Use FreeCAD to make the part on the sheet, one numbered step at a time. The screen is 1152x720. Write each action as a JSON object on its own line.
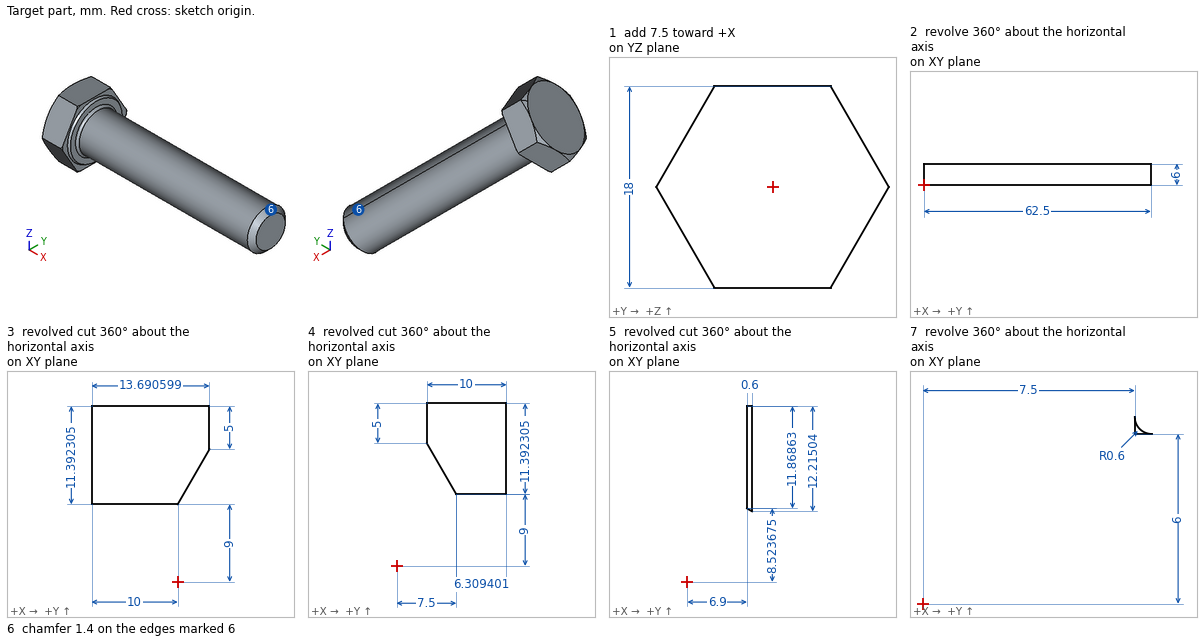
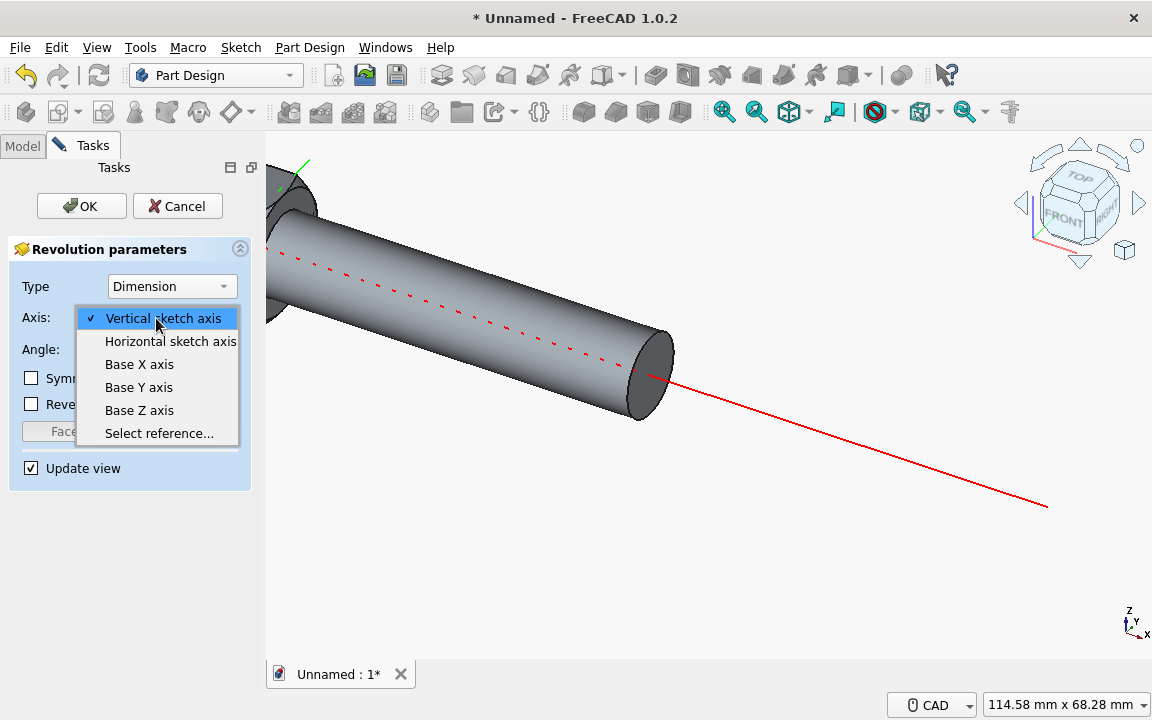
{"action": "left_click", "coordinate": [156, 342]}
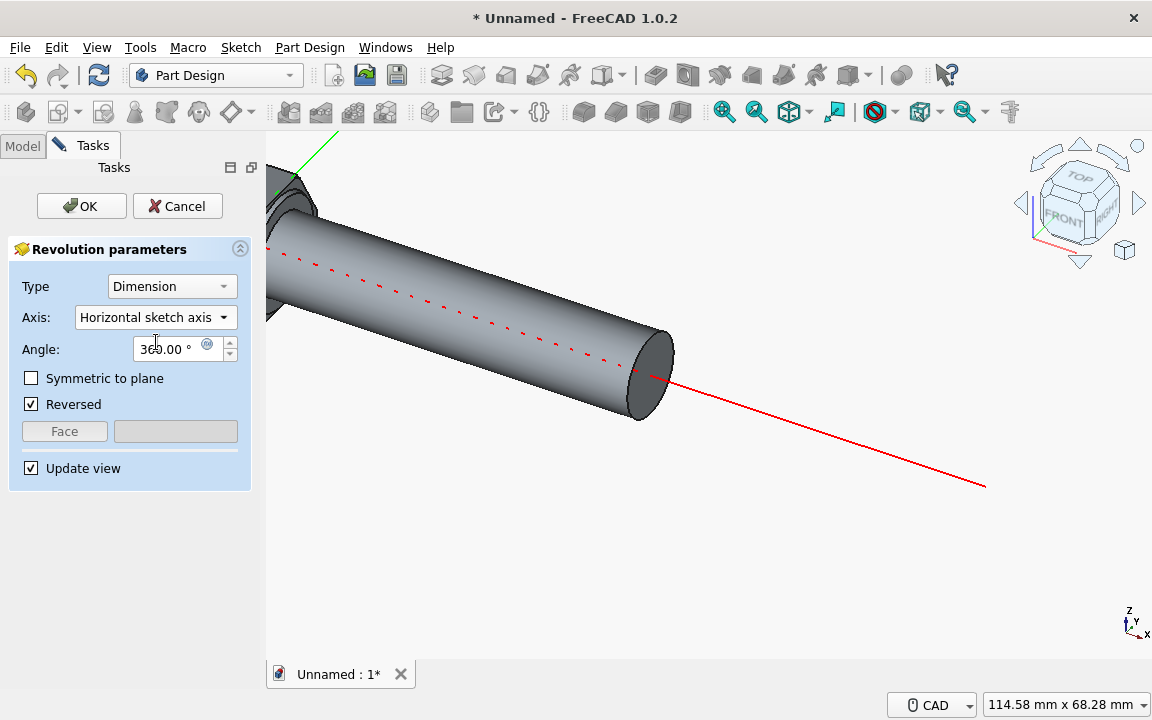
{"action": "left_click", "coordinate": [82, 206]}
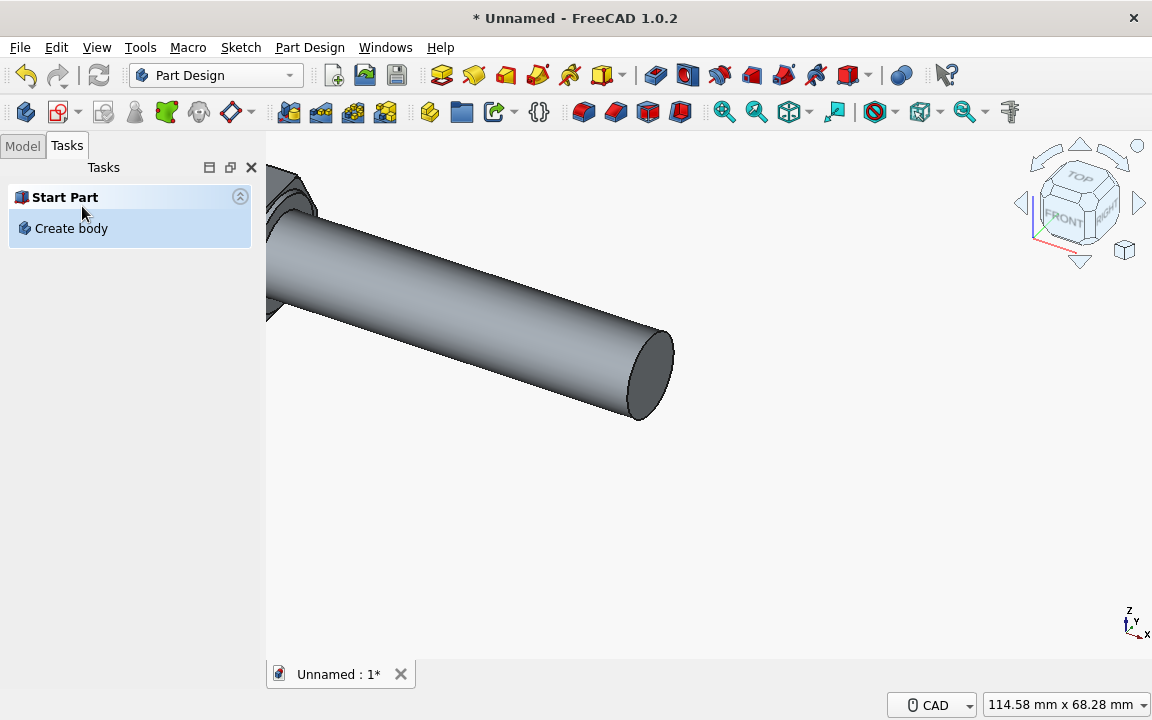
{"action": "key", "text": "v f"}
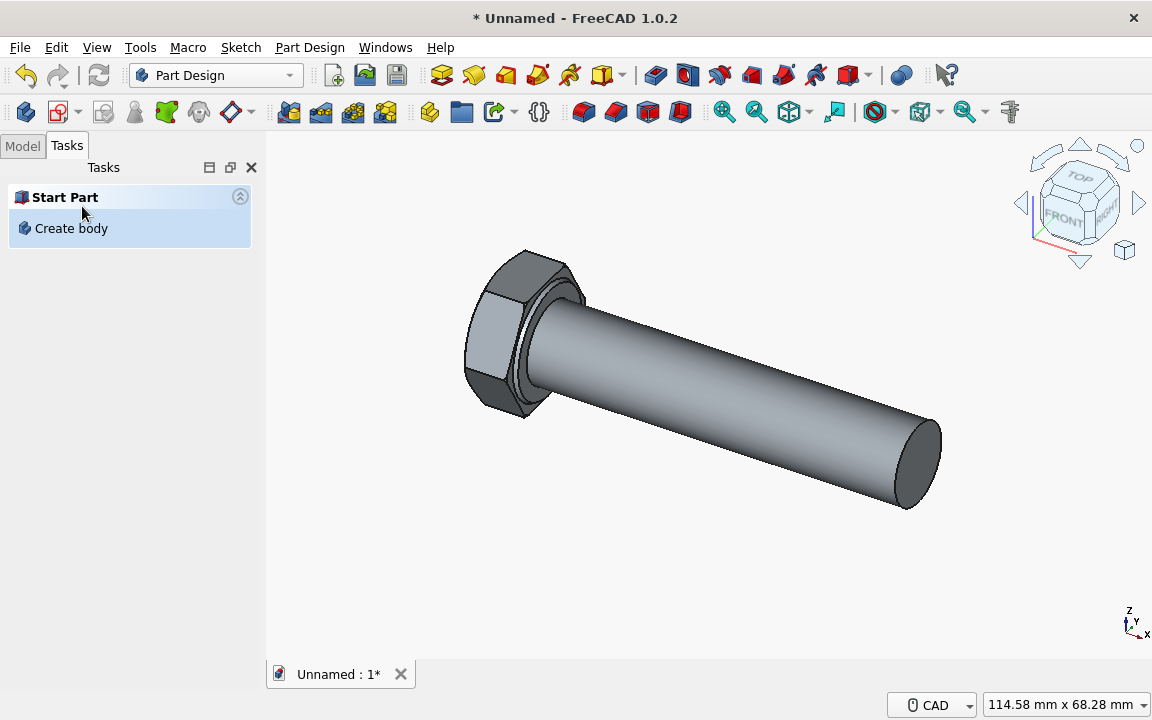
{"action": "left_click", "coordinate": [895, 486]}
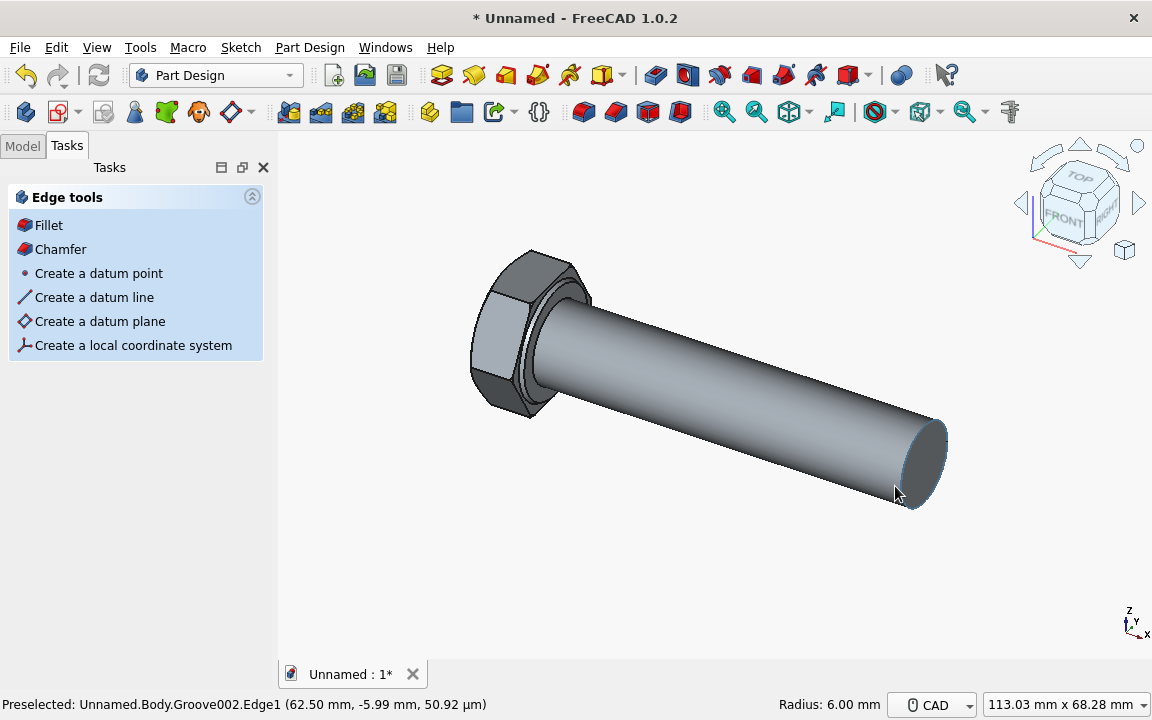
{"action": "left_click", "coordinate": [616, 112]}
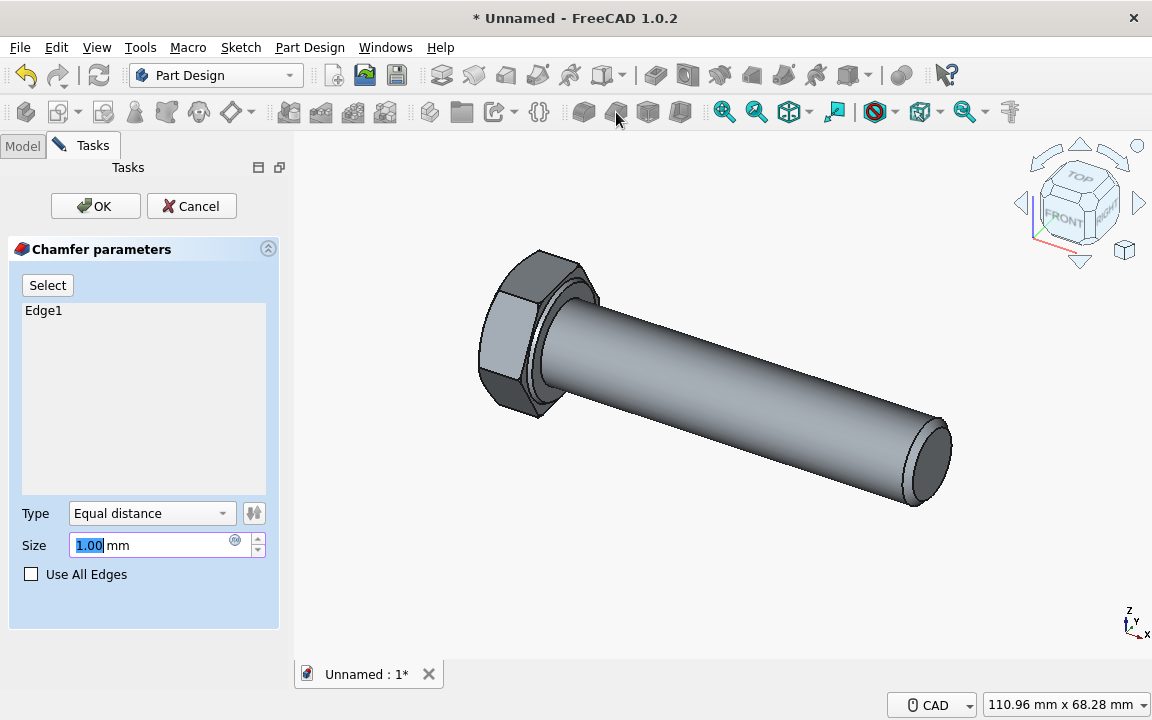
{"action": "type", "text": "1.4"}
{"action": "key", "text": "Tab"}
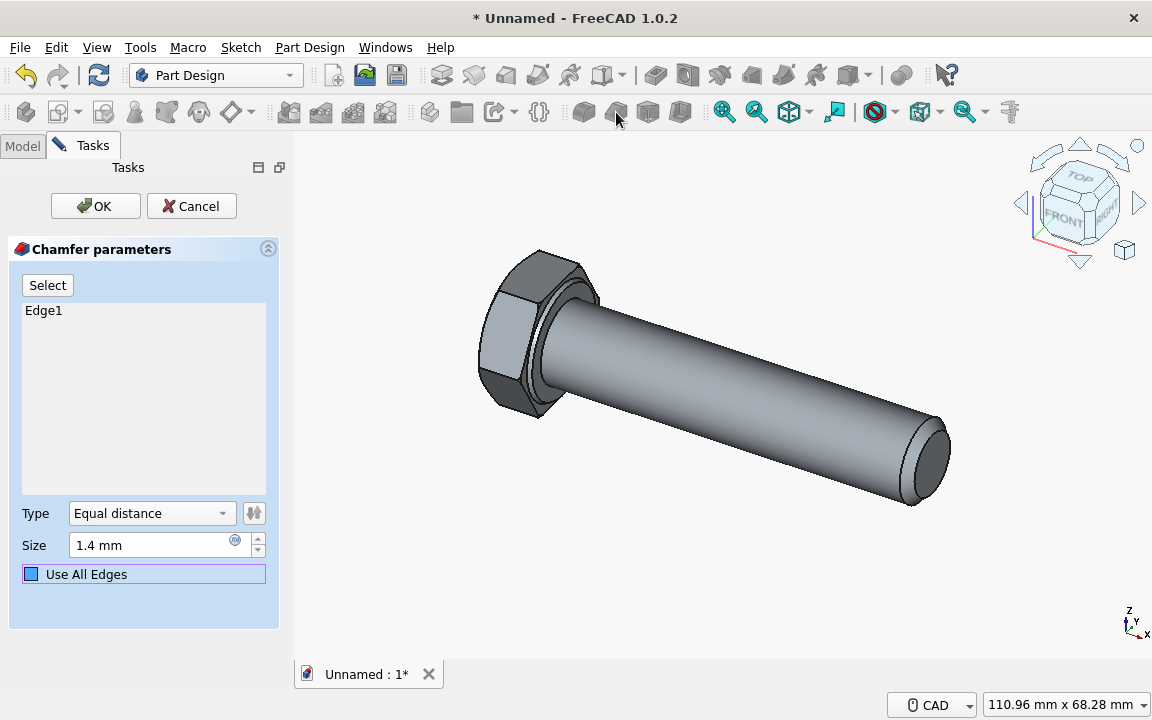
{"action": "left_click", "coordinate": [96, 206]}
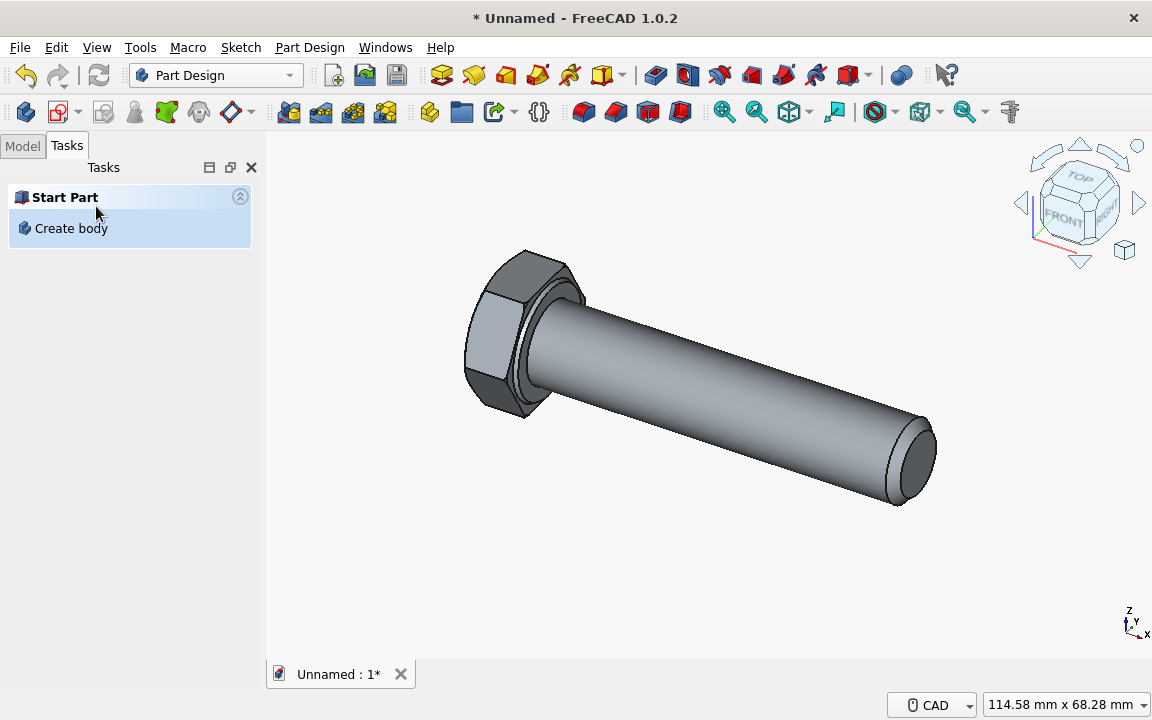
{"action": "left_click", "coordinate": [58, 112]}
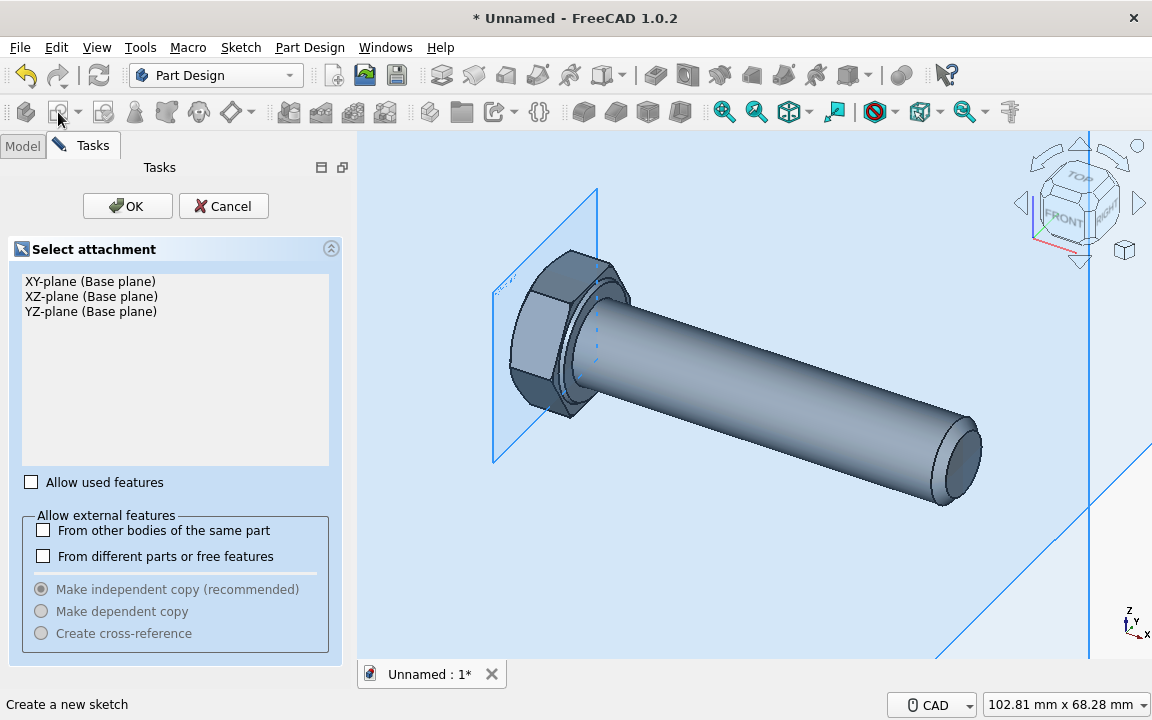
{"action": "left_click", "coordinate": [82, 282]}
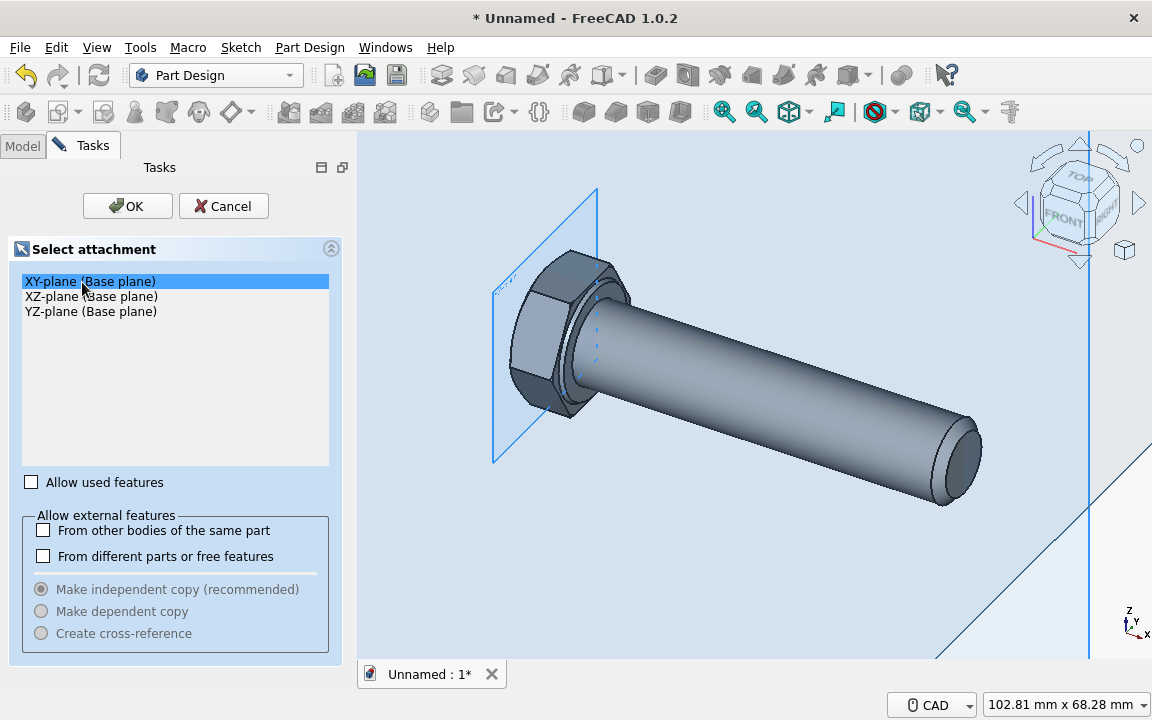
{"action": "left_click", "coordinate": [128, 206]}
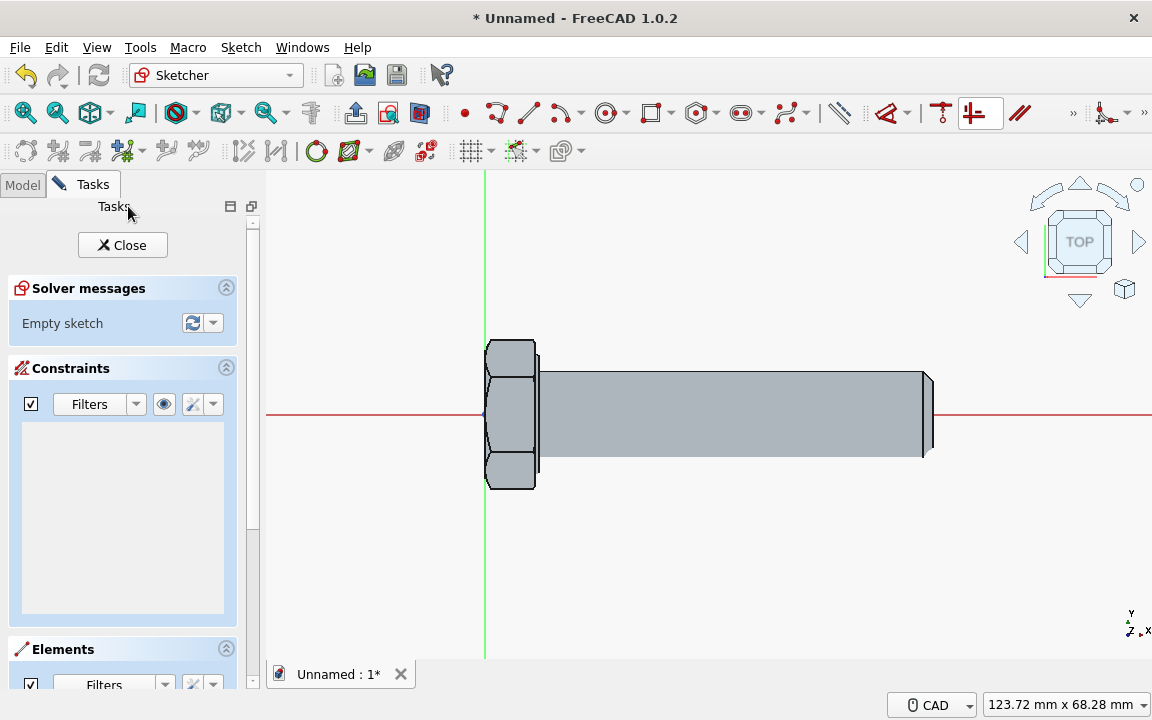
{"action": "left_click", "coordinate": [420, 114]}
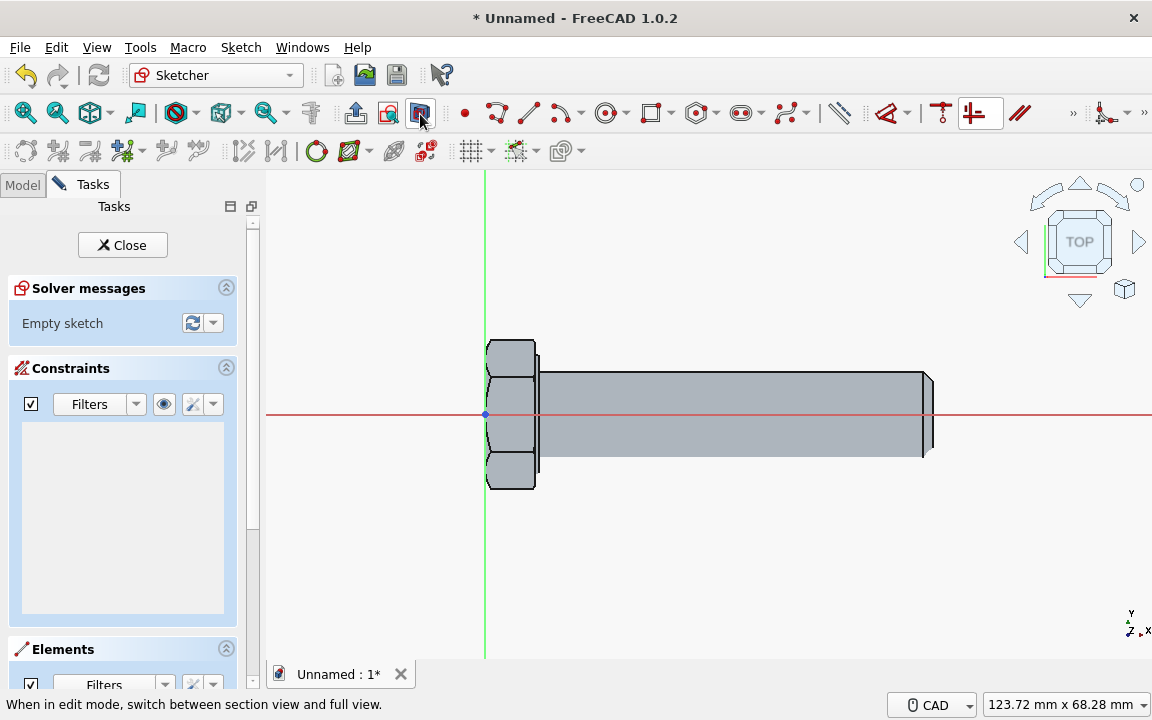
{"action": "scroll", "coordinate": [536, 367], "scroll_direction": "up", "scroll_amount": 15}